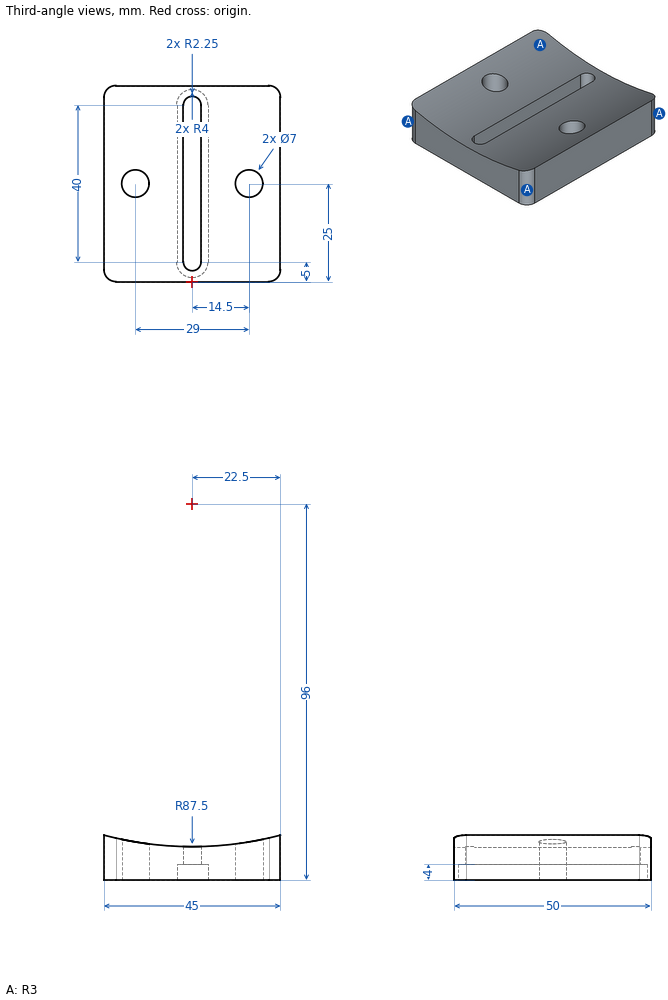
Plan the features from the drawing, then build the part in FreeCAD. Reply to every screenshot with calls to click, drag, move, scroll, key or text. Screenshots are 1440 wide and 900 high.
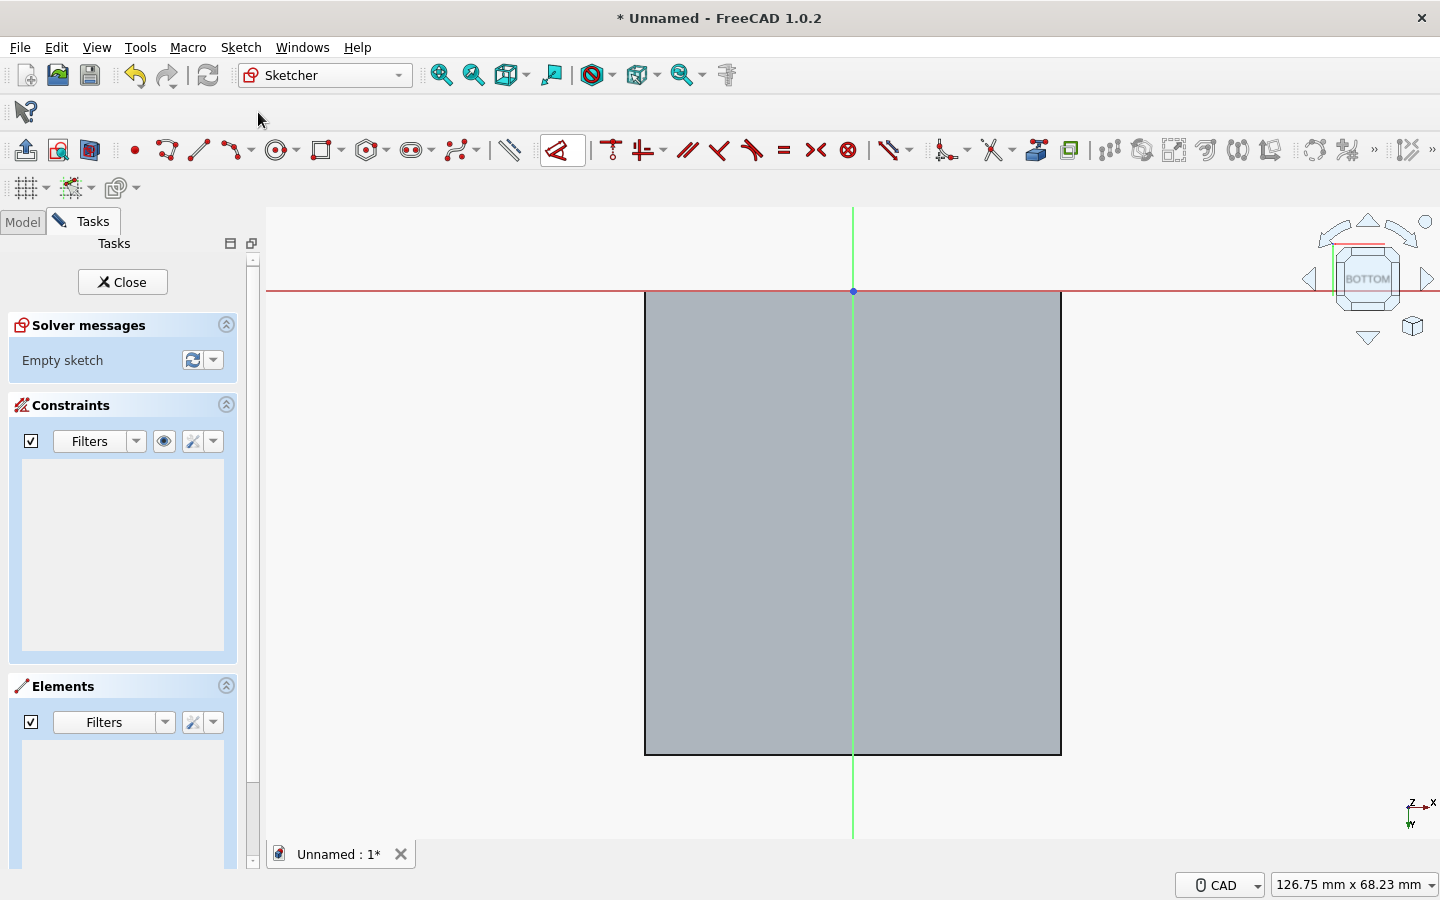
scroll(992, 235, up, 2)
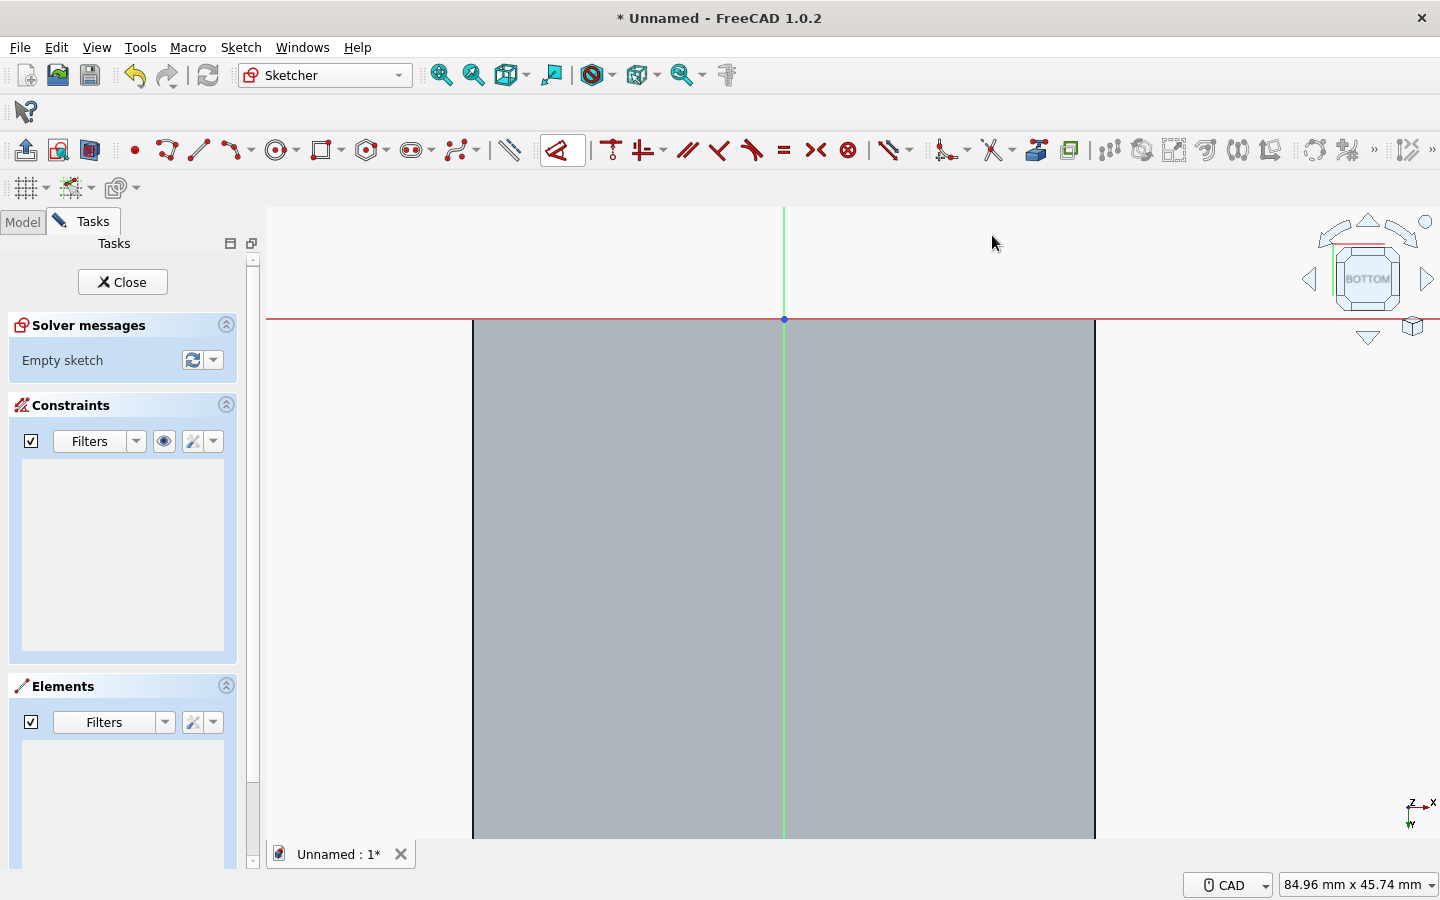
click(276, 150)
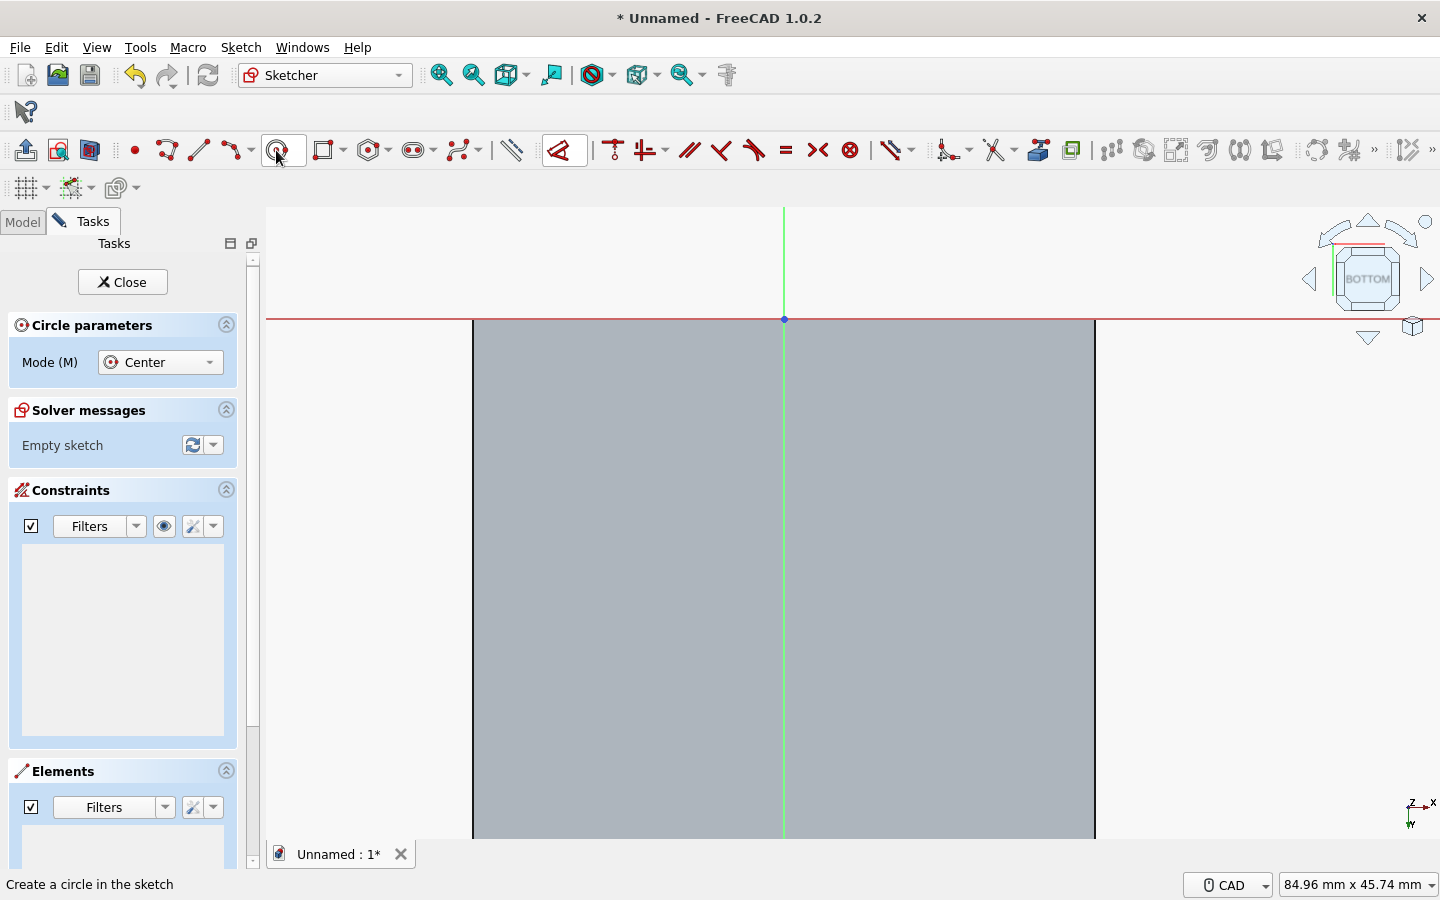
click(985, 665)
click(1019, 630)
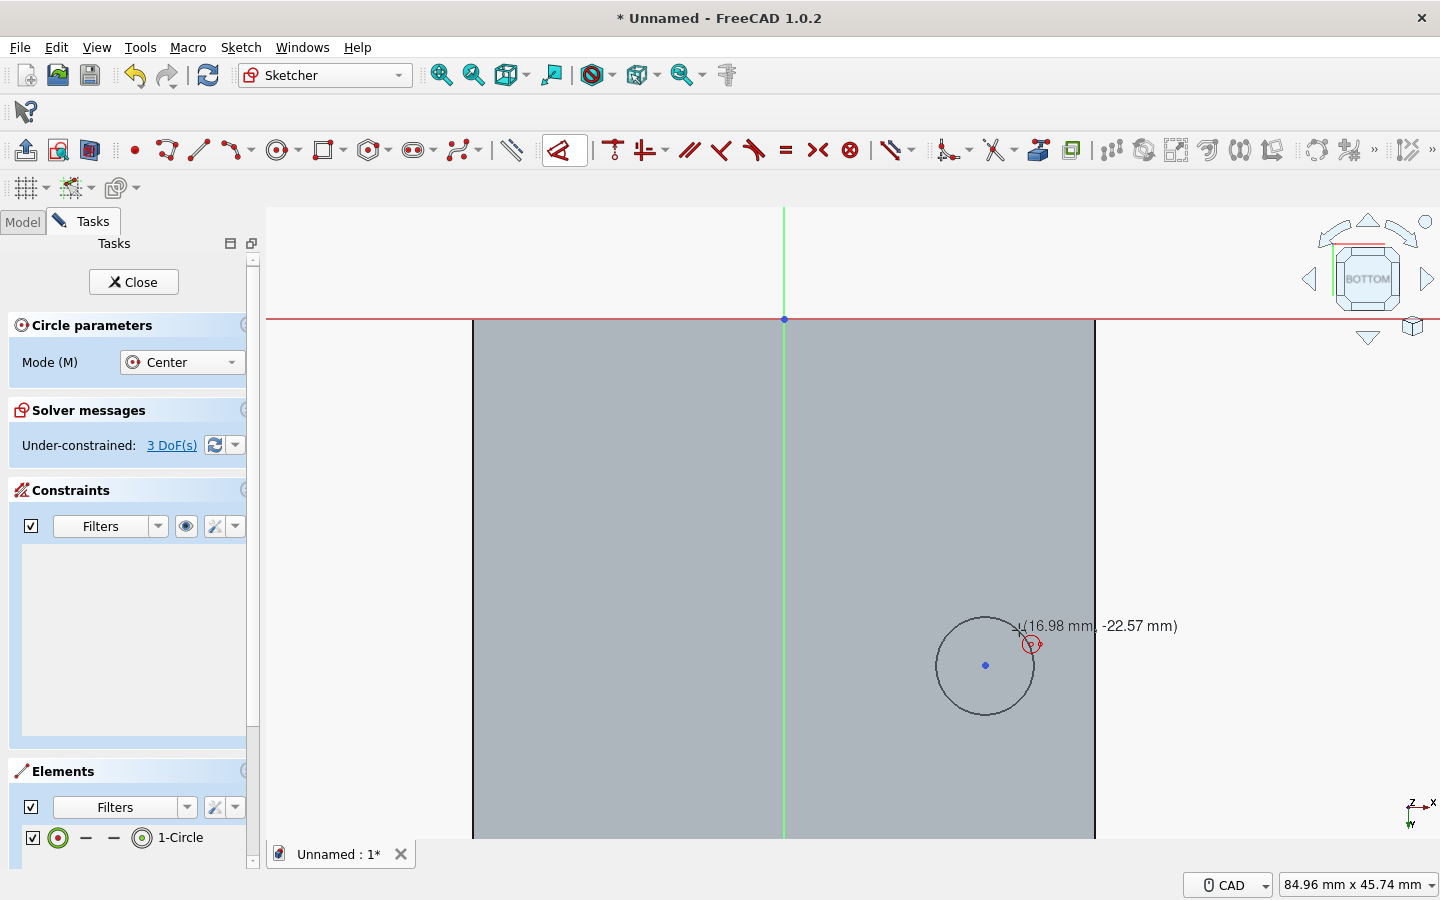
click(584, 665)
click(618, 630)
key(Escape)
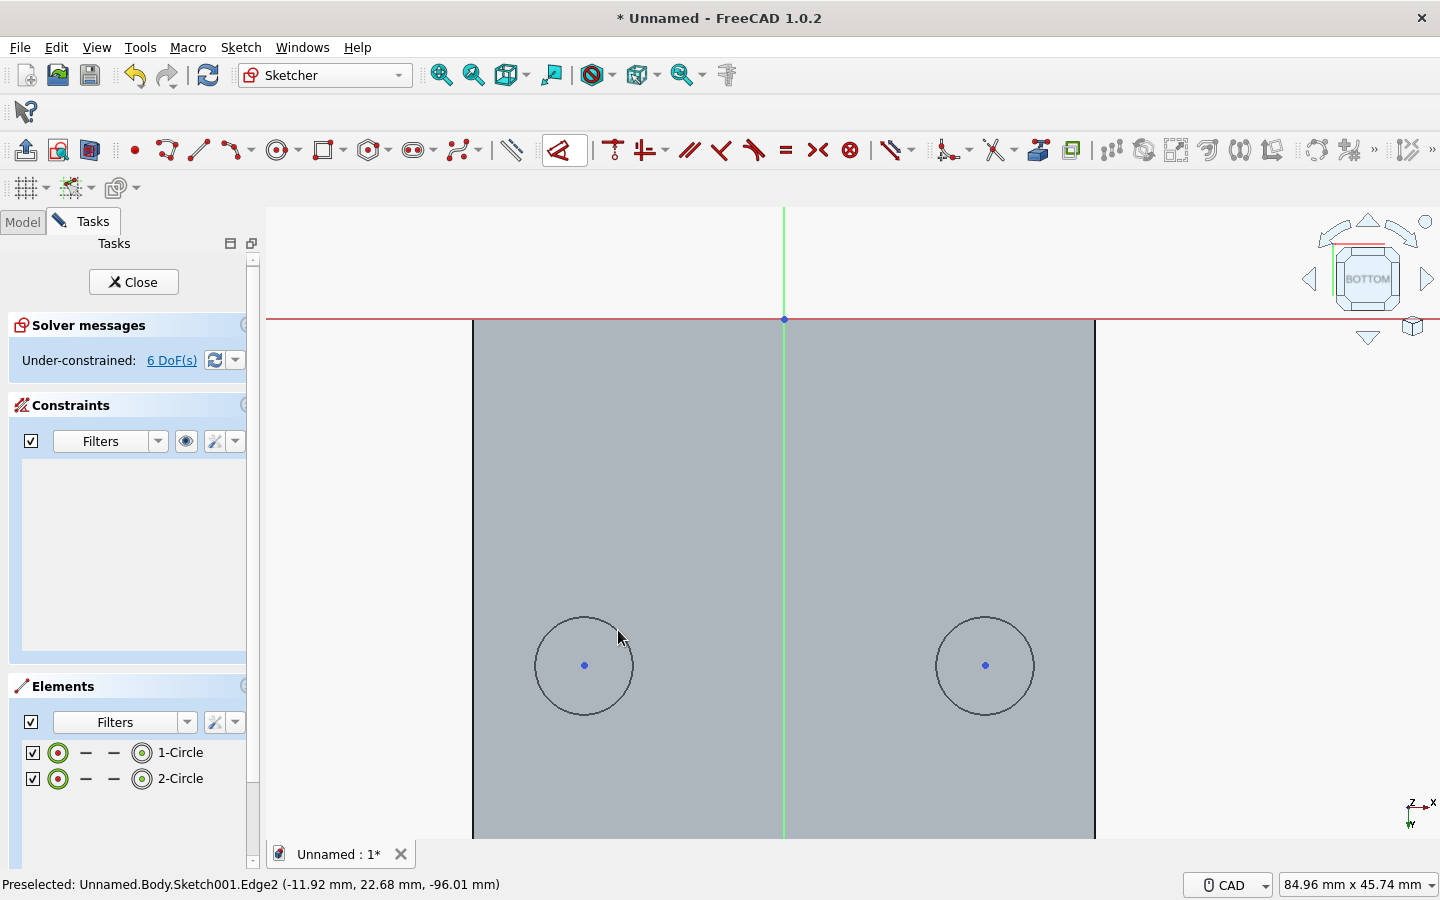
click(1019, 631)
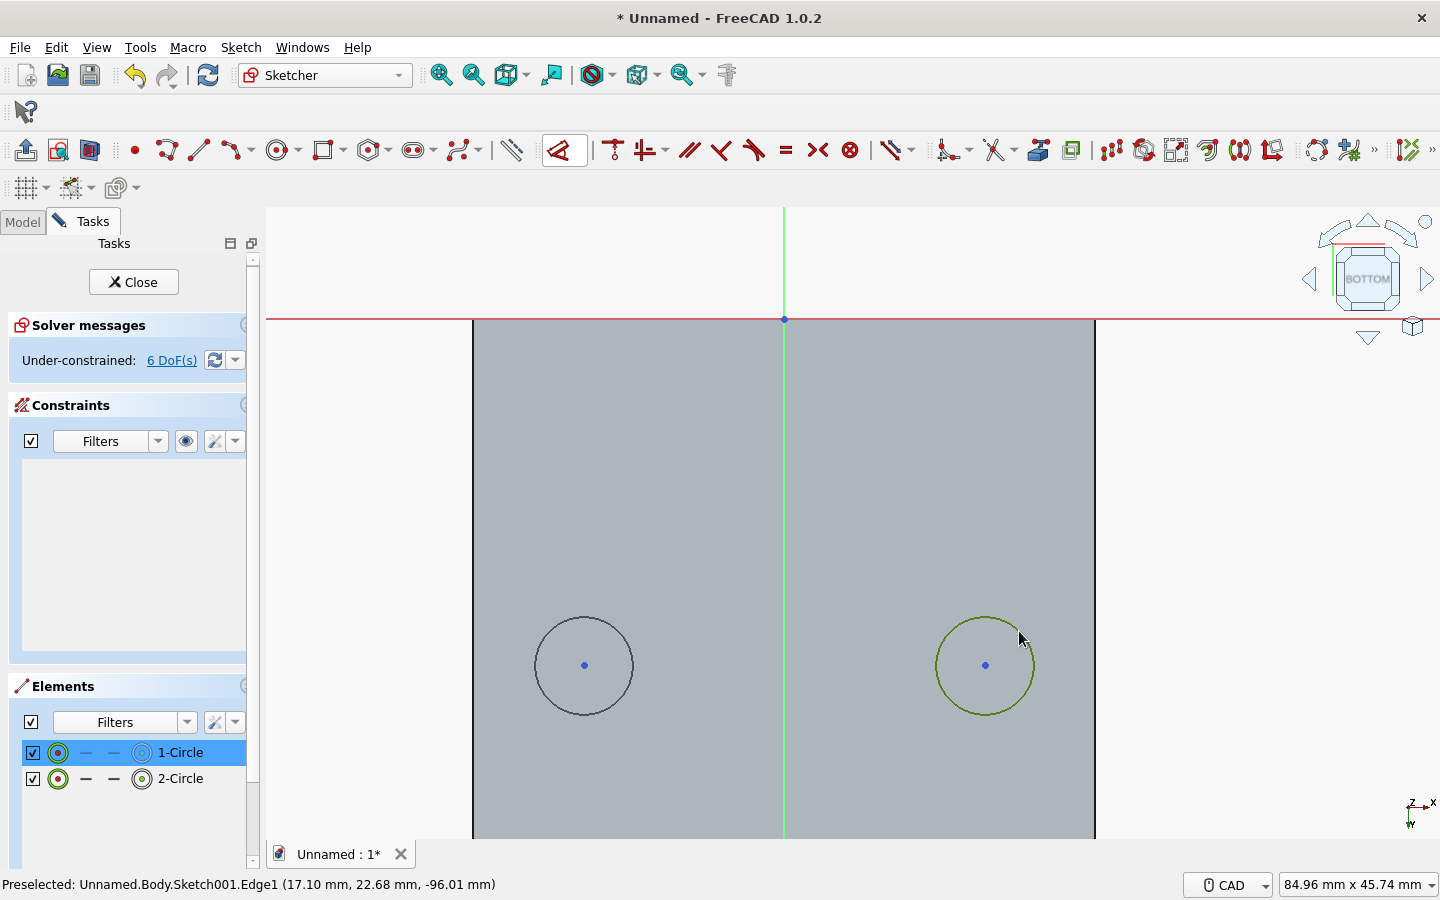
click(618, 631)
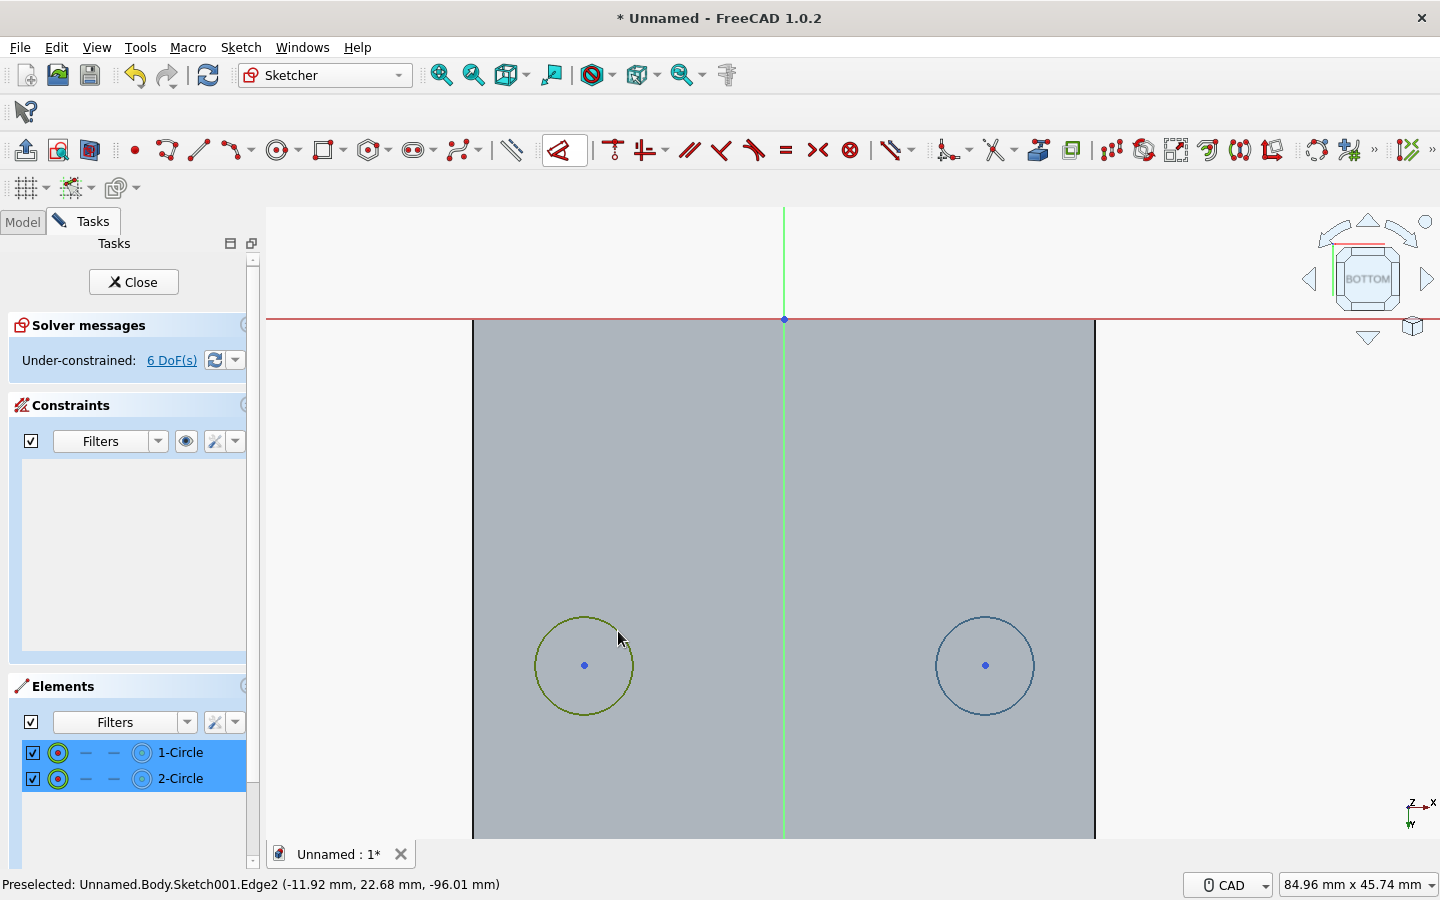
click(786, 150)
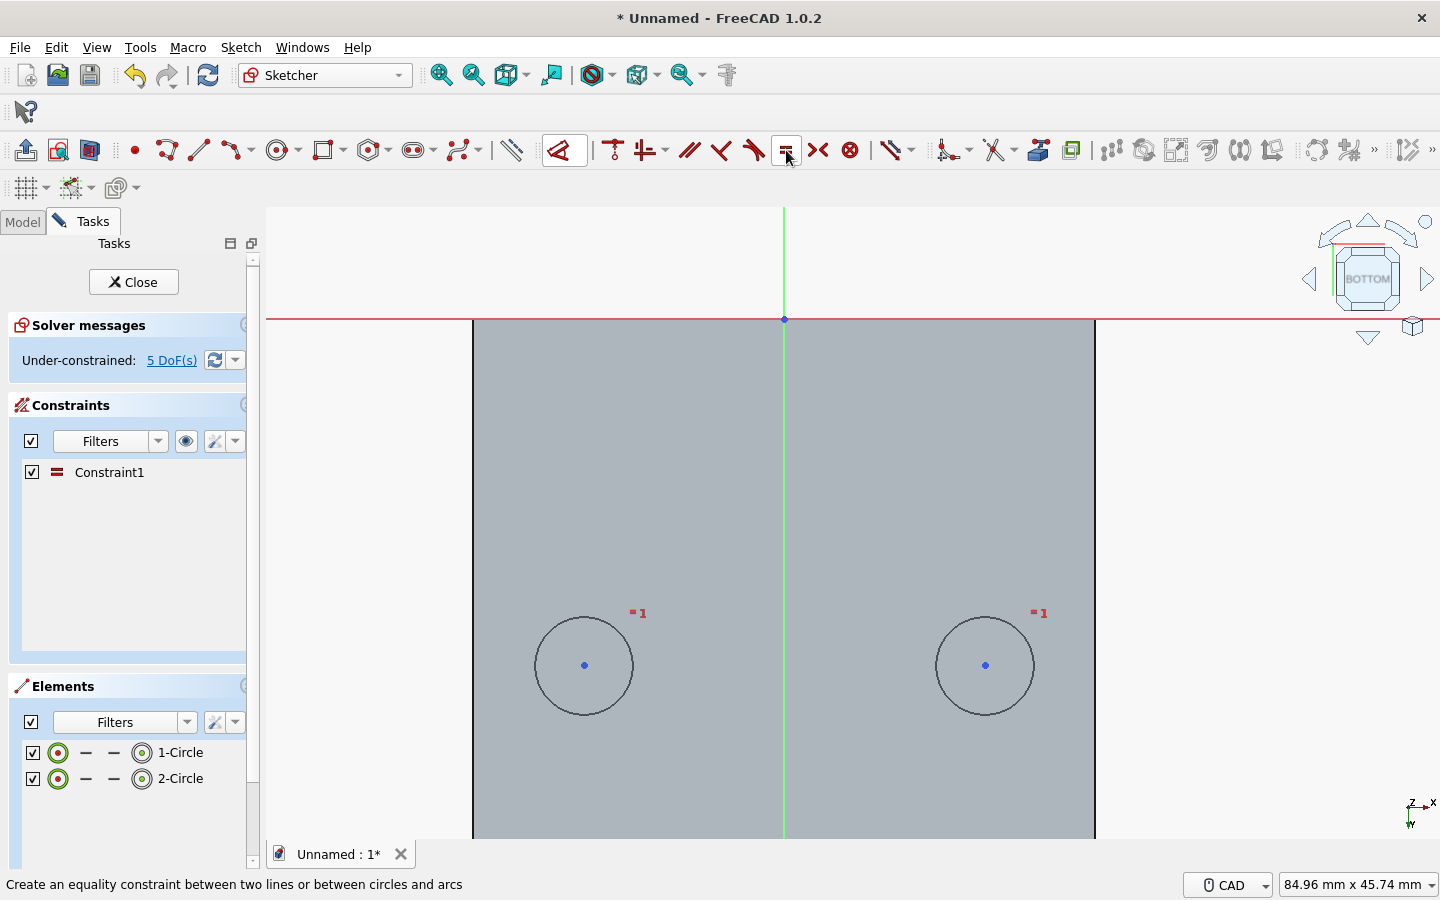
click(985, 666)